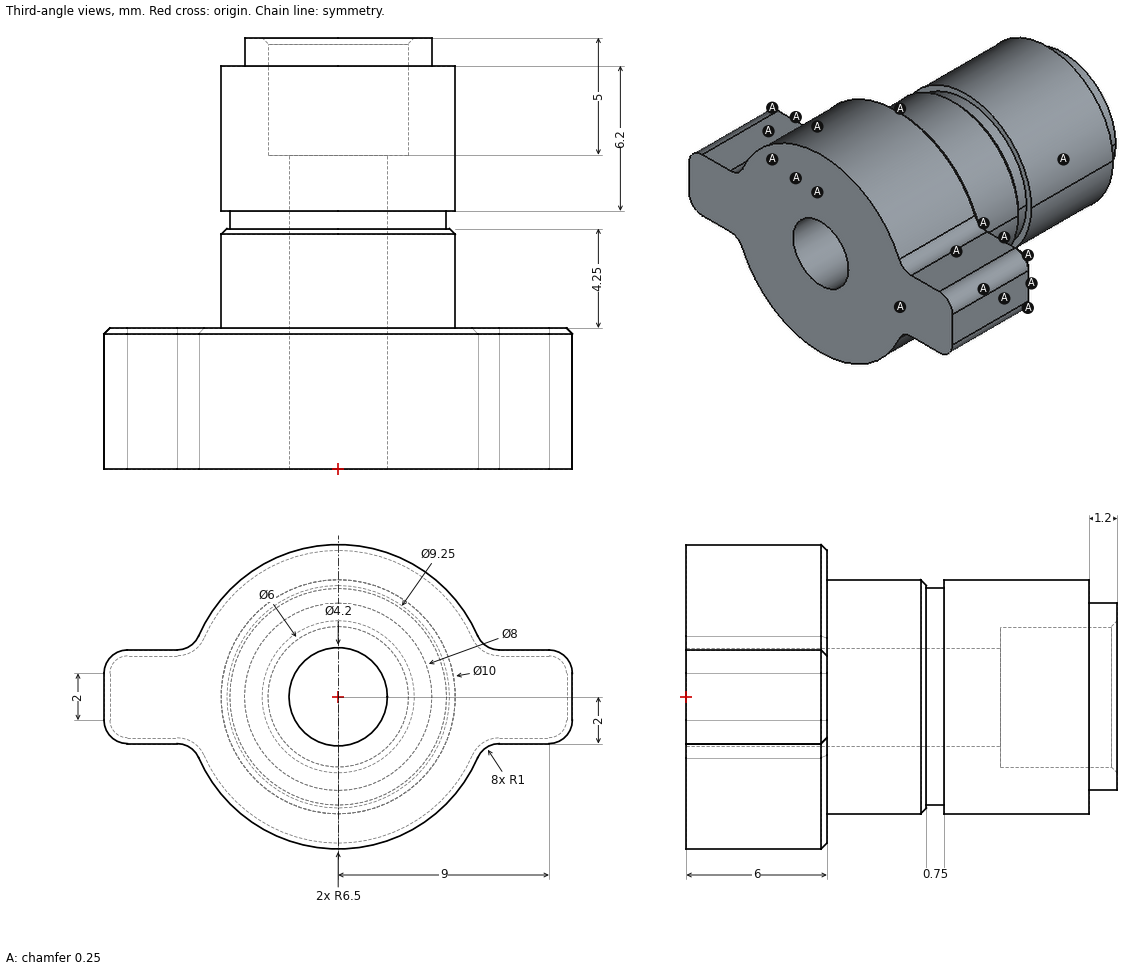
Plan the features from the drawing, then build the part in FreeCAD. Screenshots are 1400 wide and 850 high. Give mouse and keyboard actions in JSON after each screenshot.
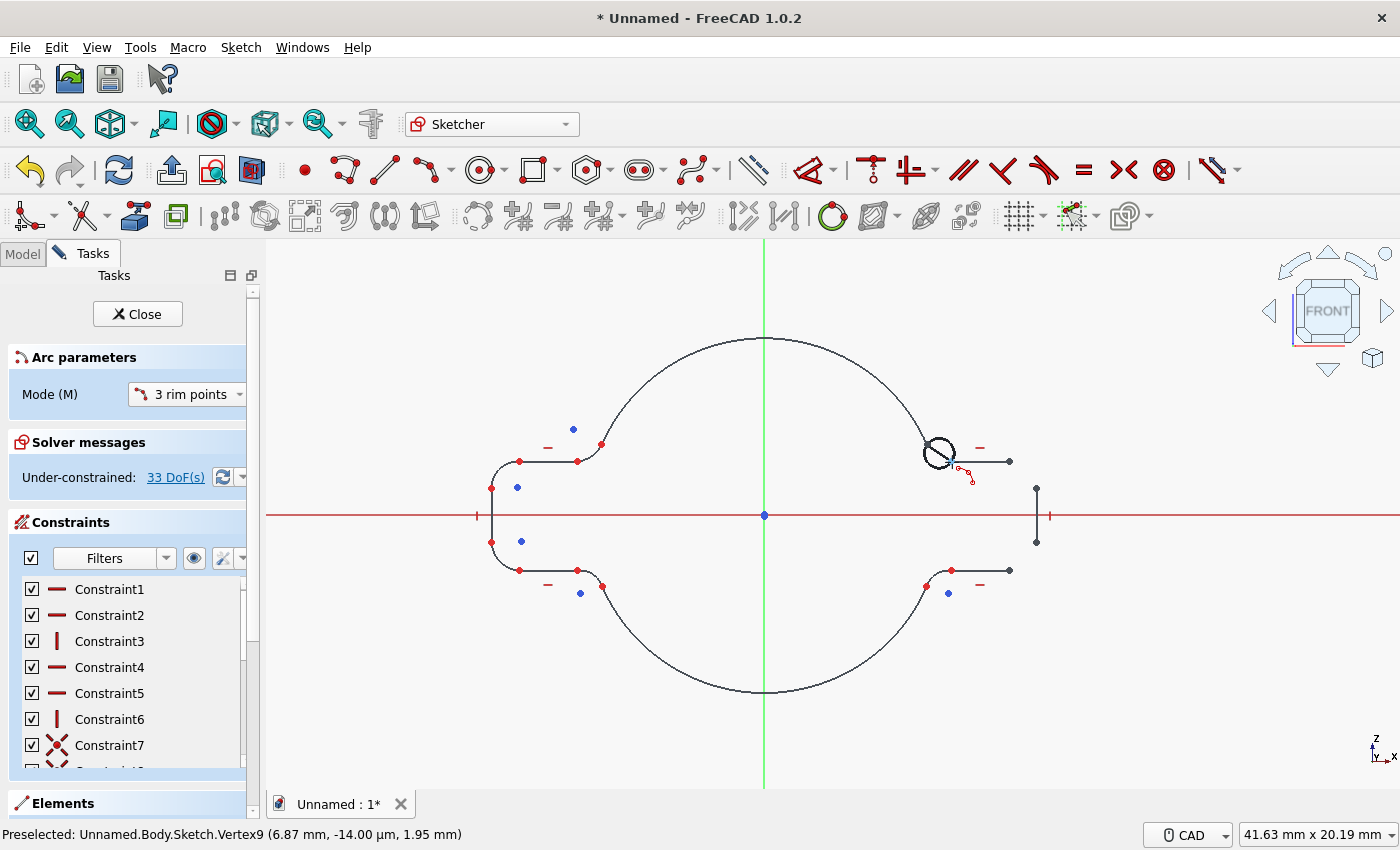
{"action": "scroll", "coordinate": [937, 456], "scroll_direction": "up", "scroll_amount": 7}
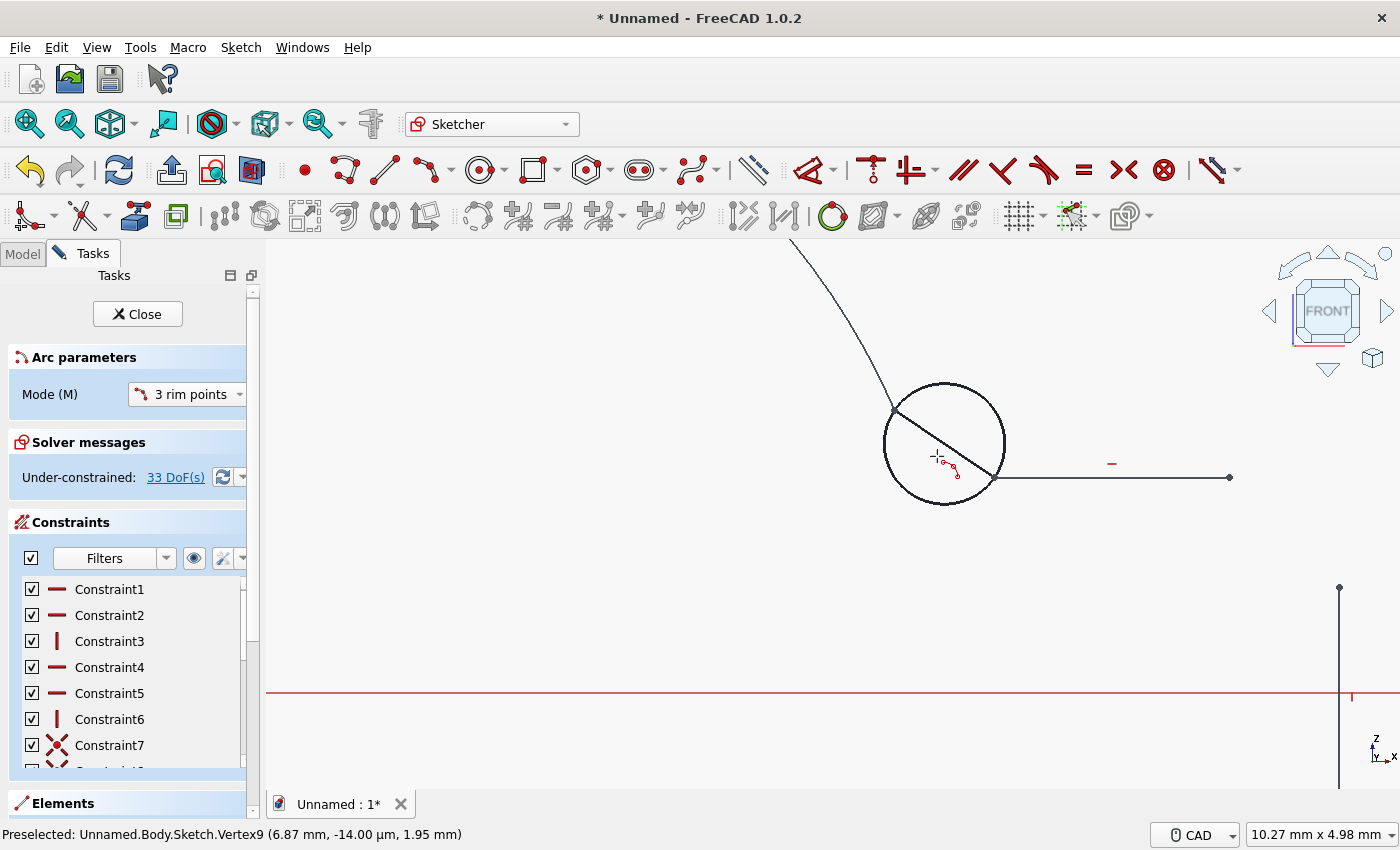
{"action": "left_click", "coordinate": [934, 454]}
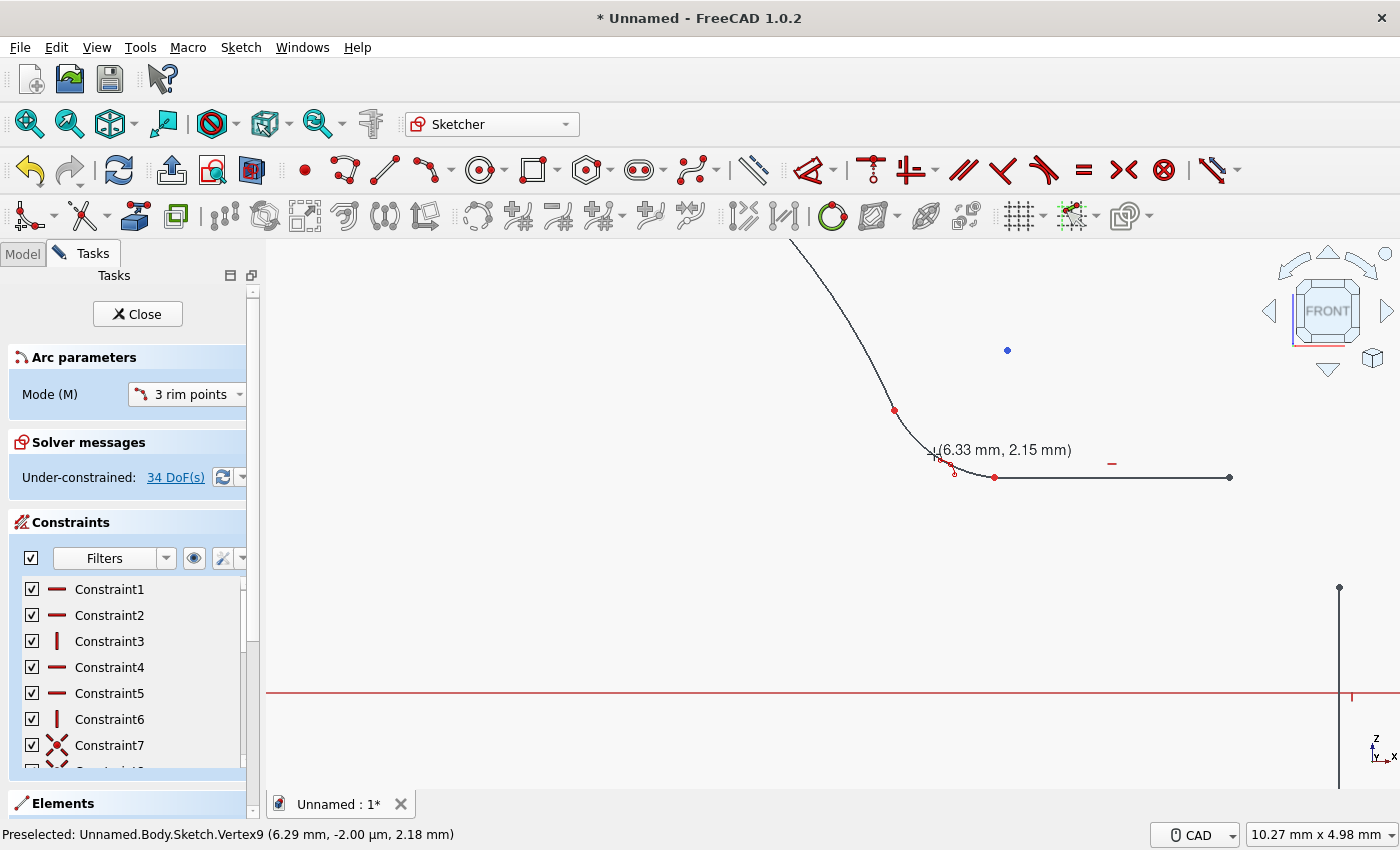
{"action": "scroll", "coordinate": [938, 456], "scroll_direction": "down", "scroll_amount": 7}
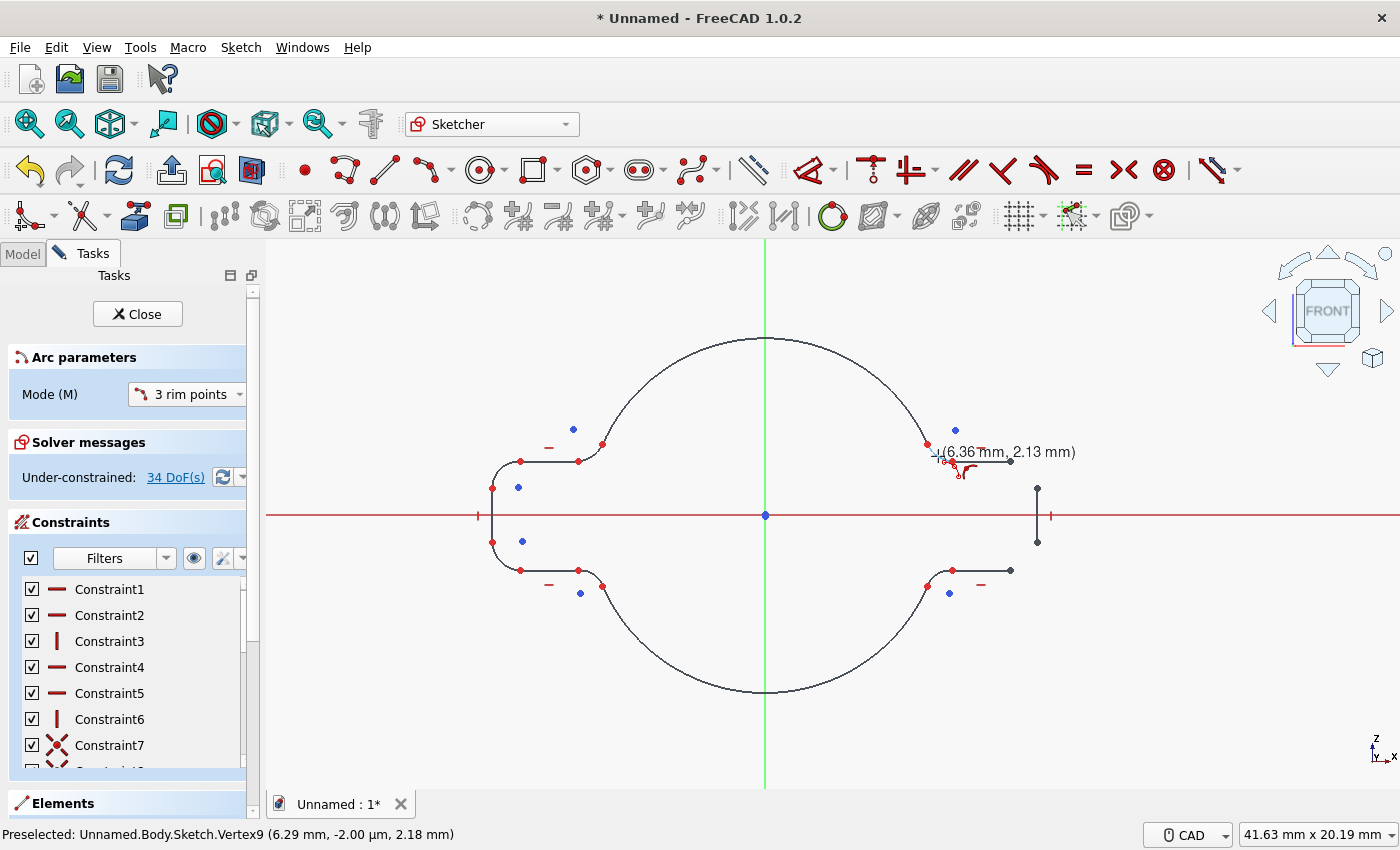
{"action": "left_click", "coordinate": [1010, 462]}
{"action": "left_click", "coordinate": [1037, 489]}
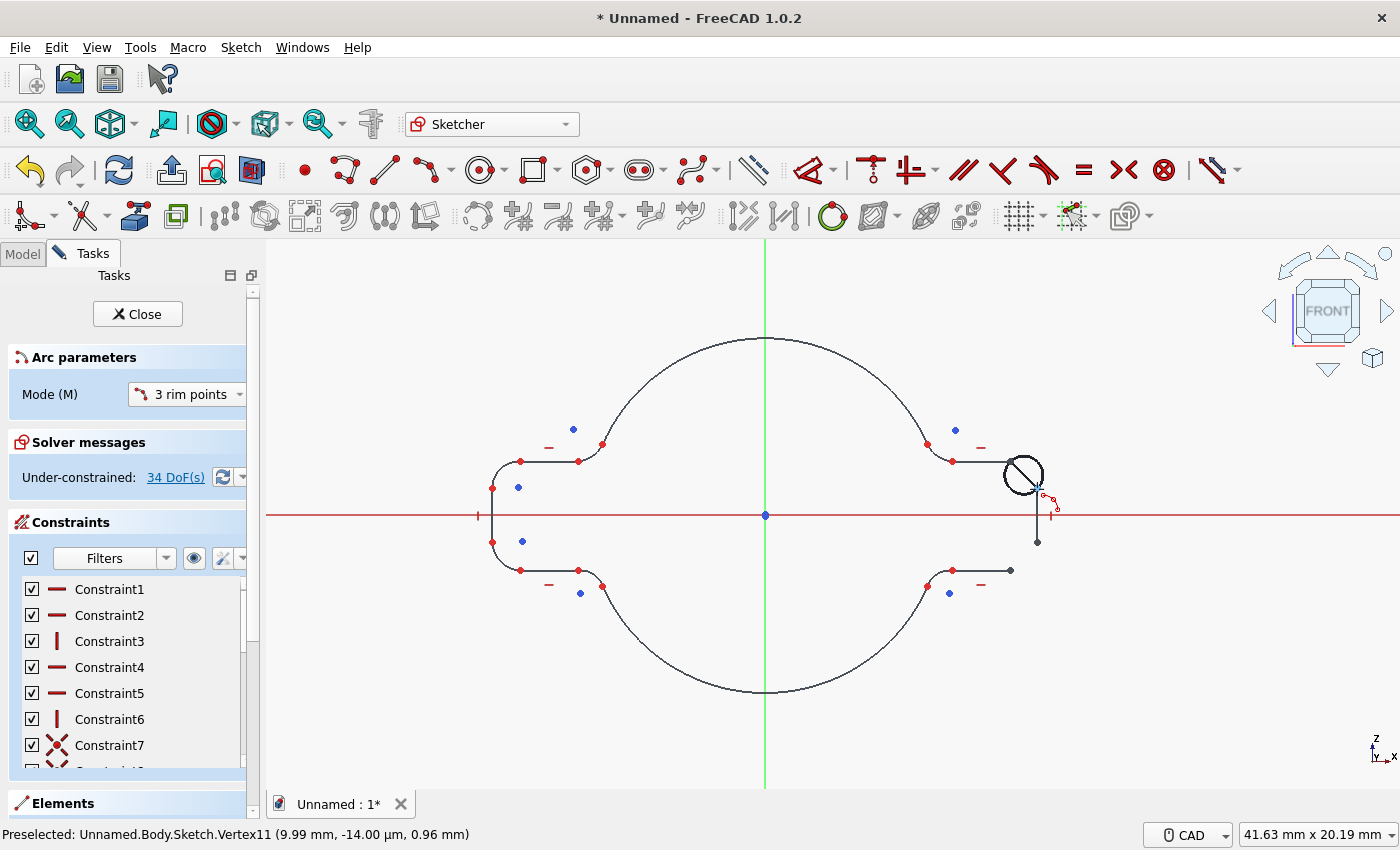
{"action": "scroll", "coordinate": [1030, 468], "scroll_direction": "up", "scroll_amount": 4}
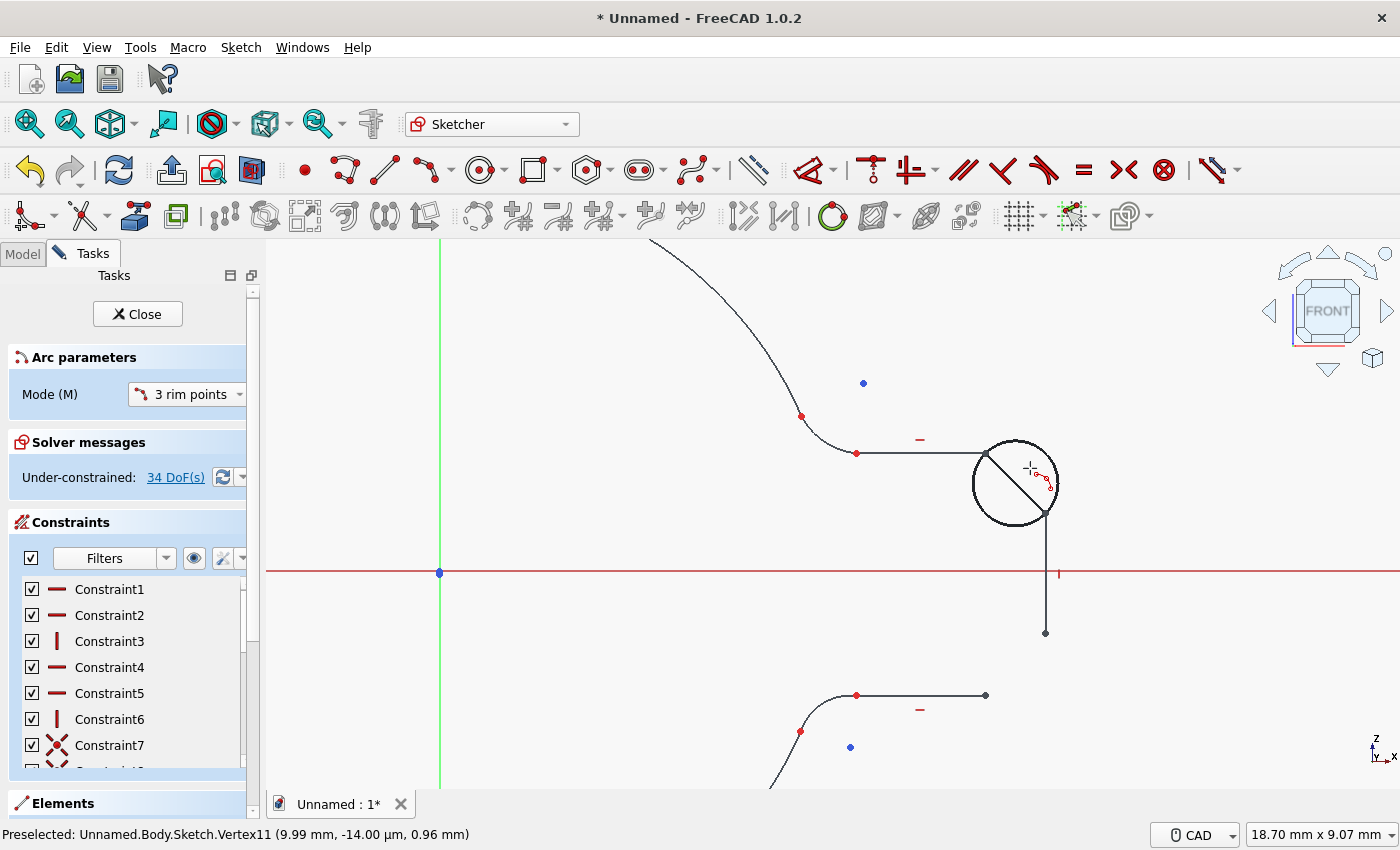
{"action": "left_click", "coordinate": [1028, 468]}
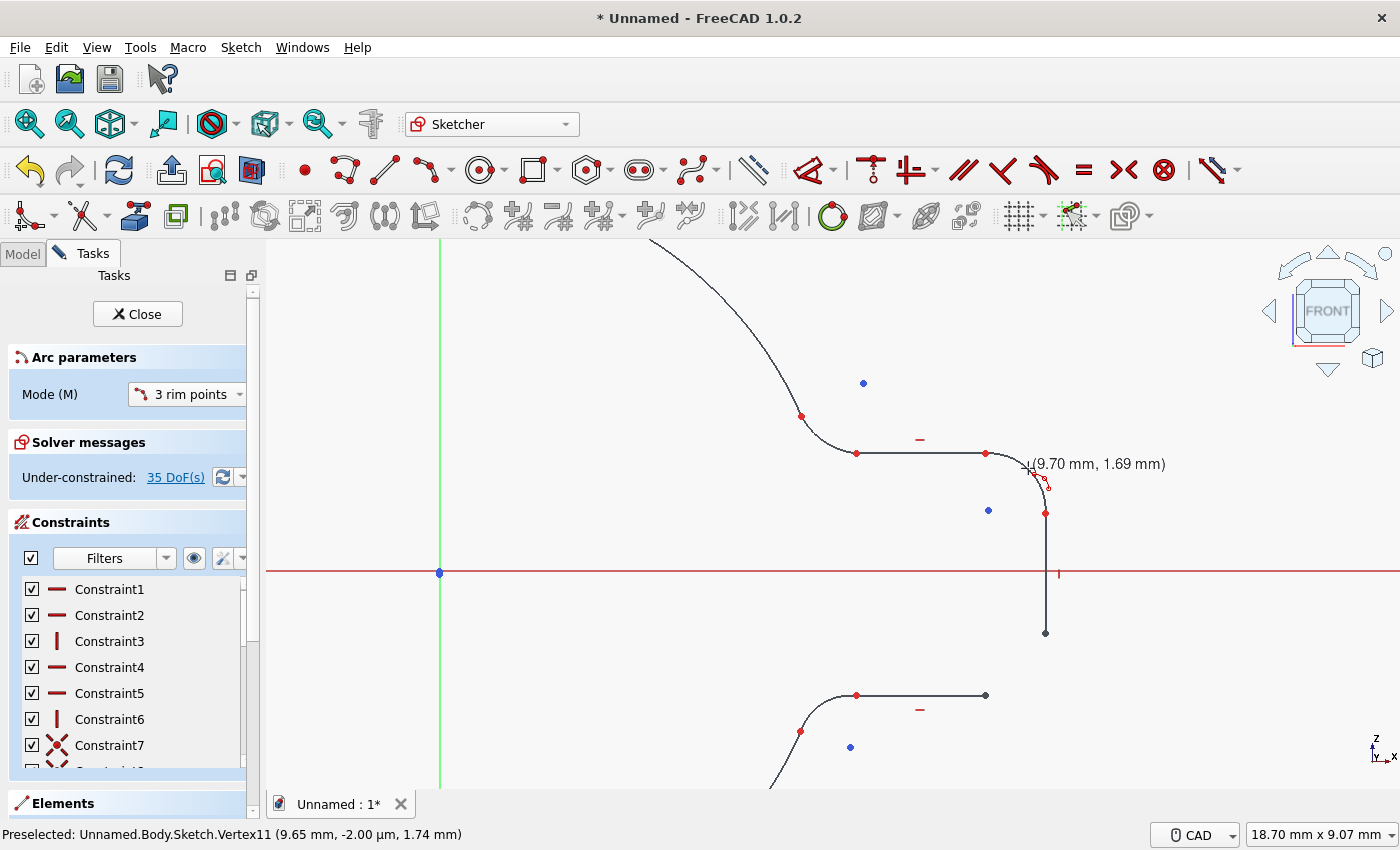
{"action": "left_click", "coordinate": [1046, 634]}
{"action": "left_click", "coordinate": [986, 696]}
{"action": "left_click", "coordinate": [1028, 675]}
{"action": "key", "text": "Escape"}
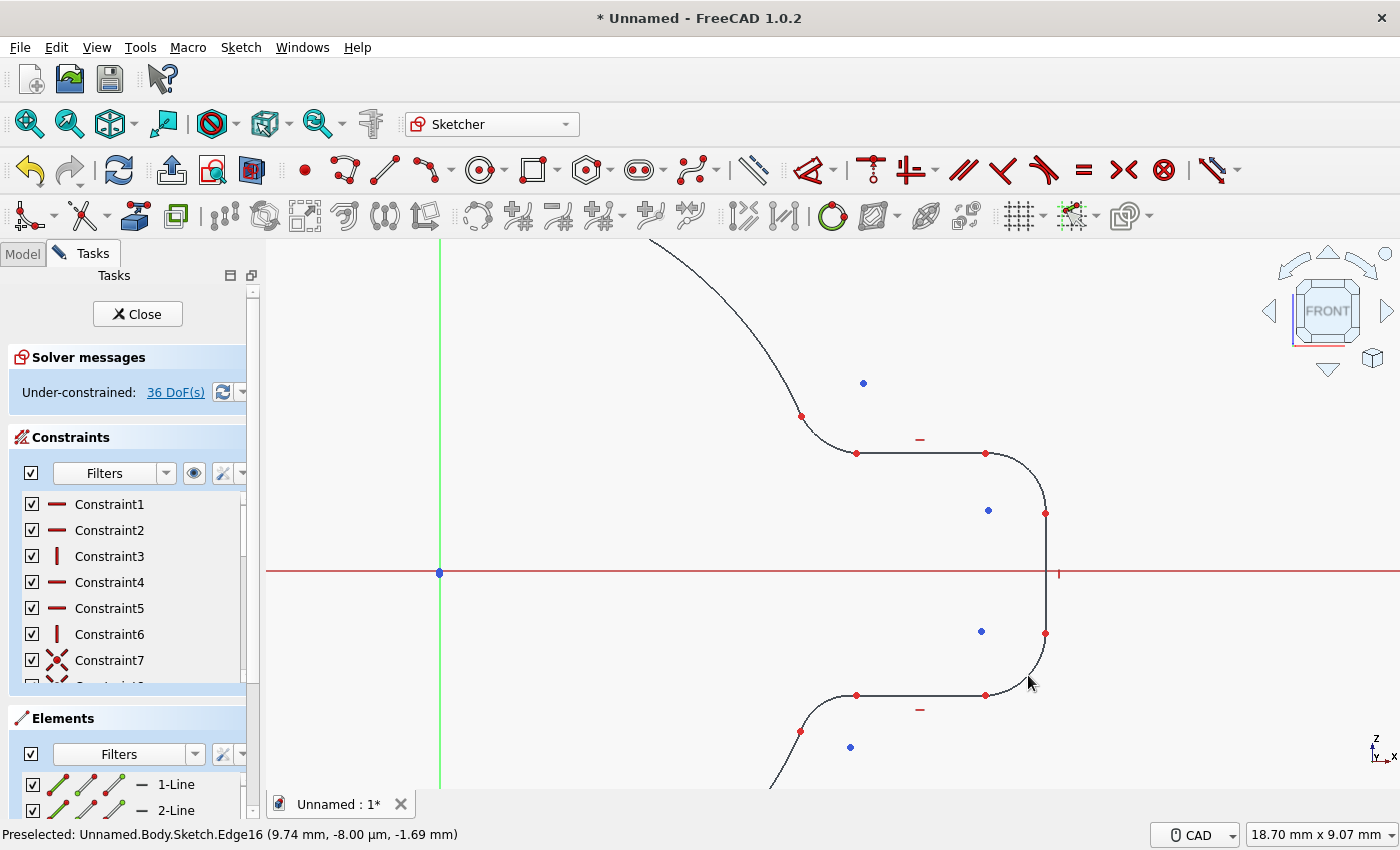
{"action": "left_click", "coordinate": [947, 696]}